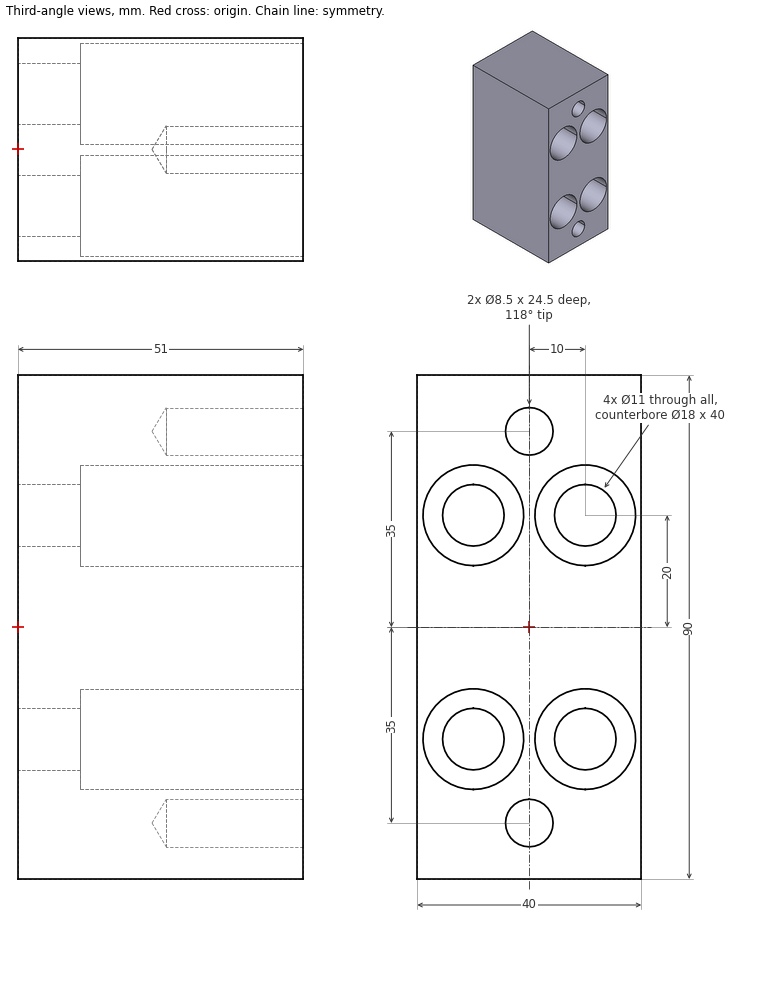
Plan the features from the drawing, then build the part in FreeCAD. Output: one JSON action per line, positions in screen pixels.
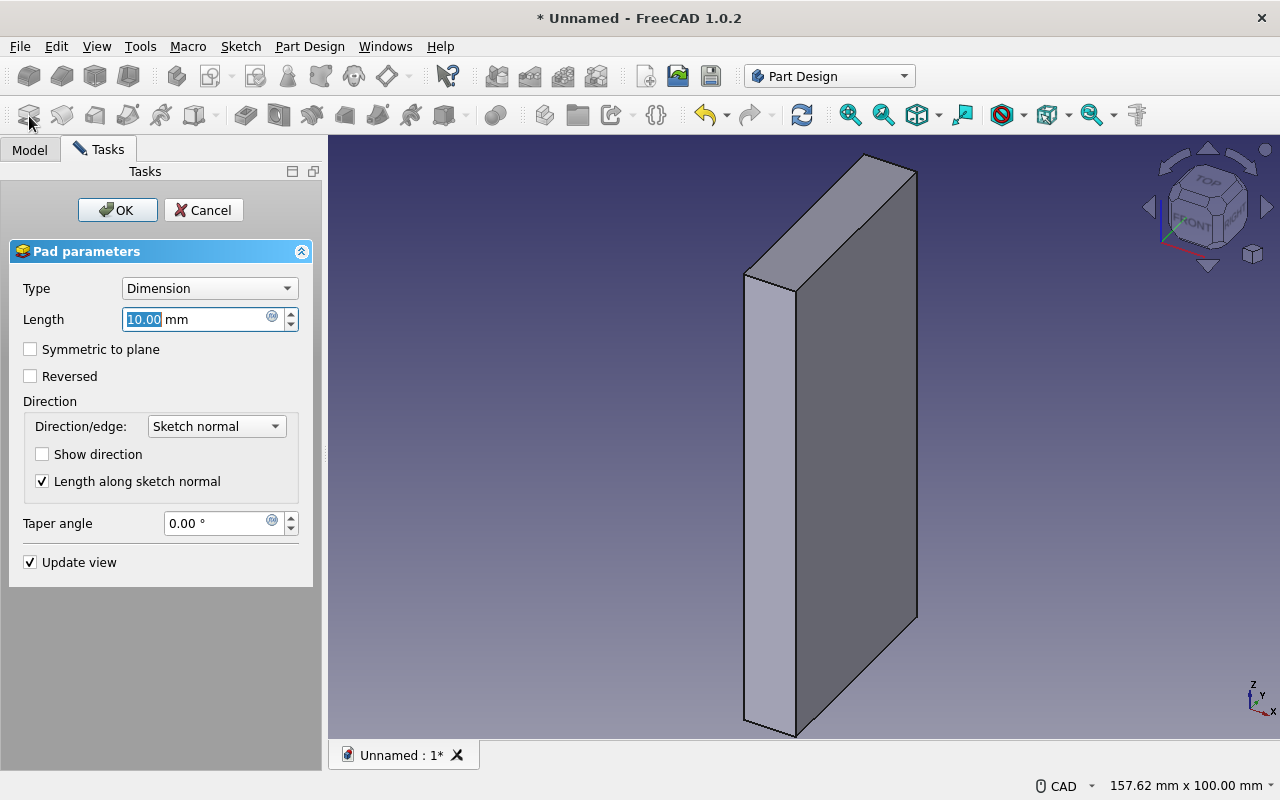
{"action": "type", "text": "51"}
{"action": "key", "text": "Tab"}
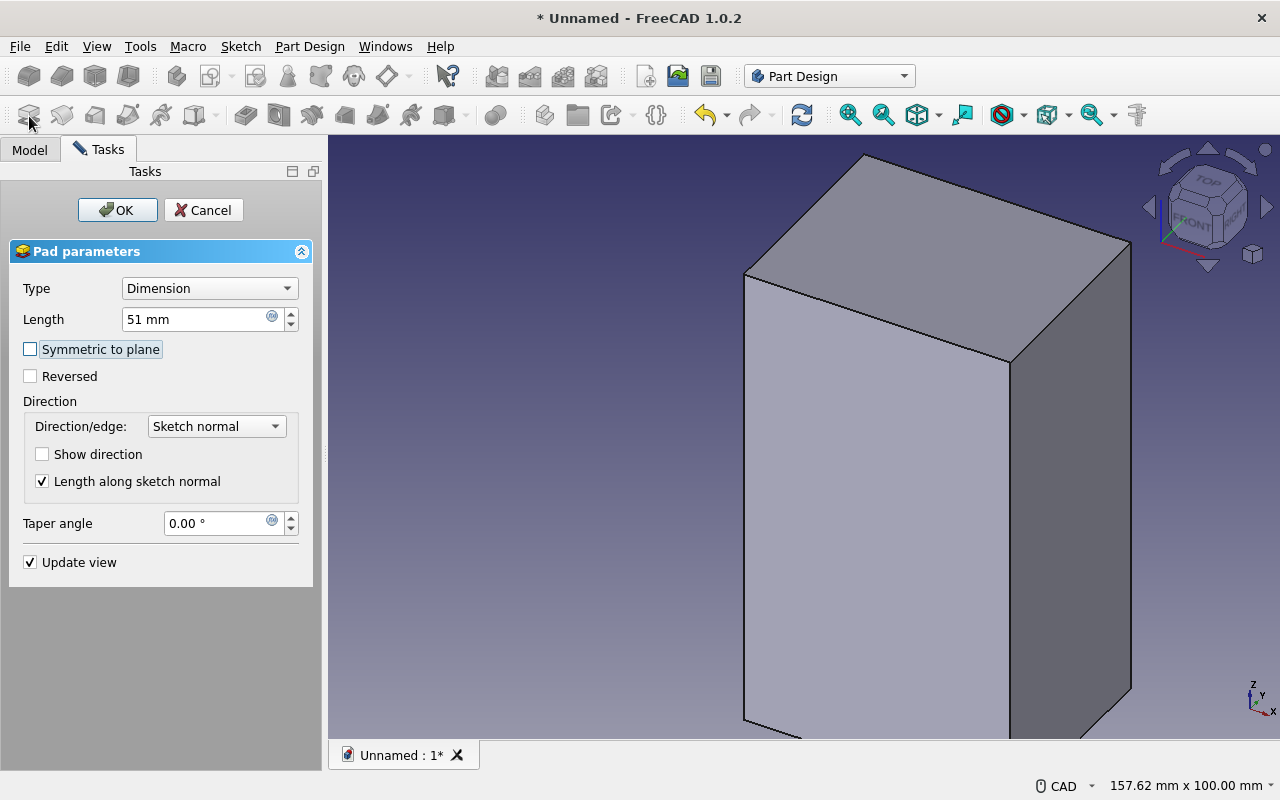
{"action": "left_click", "coordinate": [118, 210]}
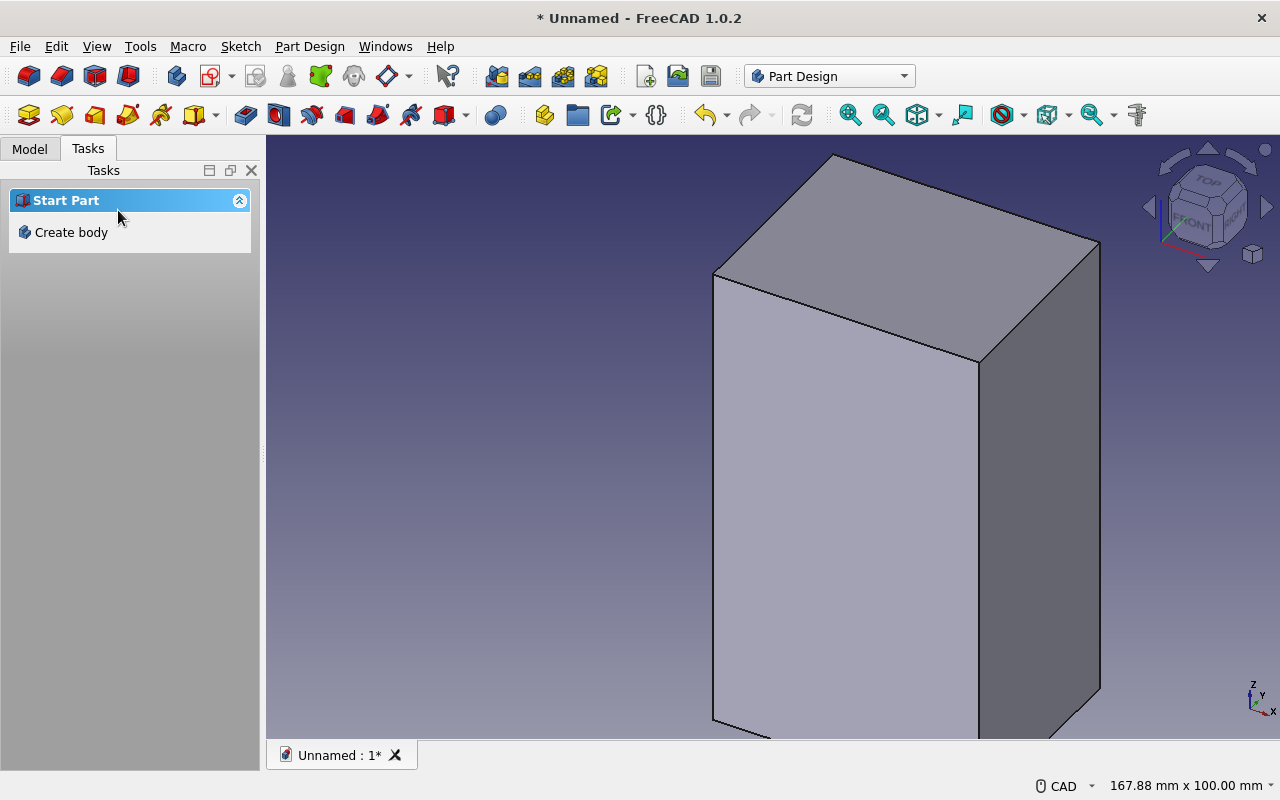
{"action": "left_click", "coordinate": [851, 116]}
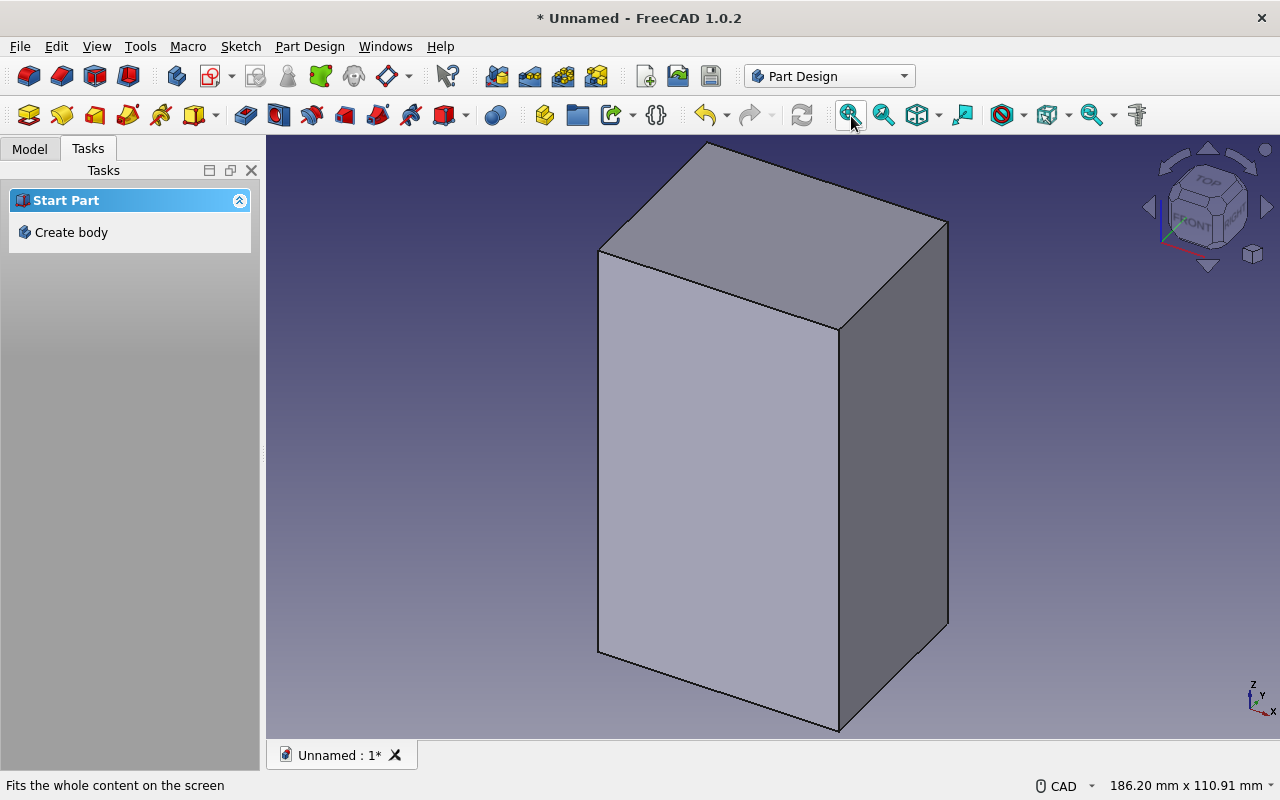
{"action": "left_click", "coordinate": [893, 533]}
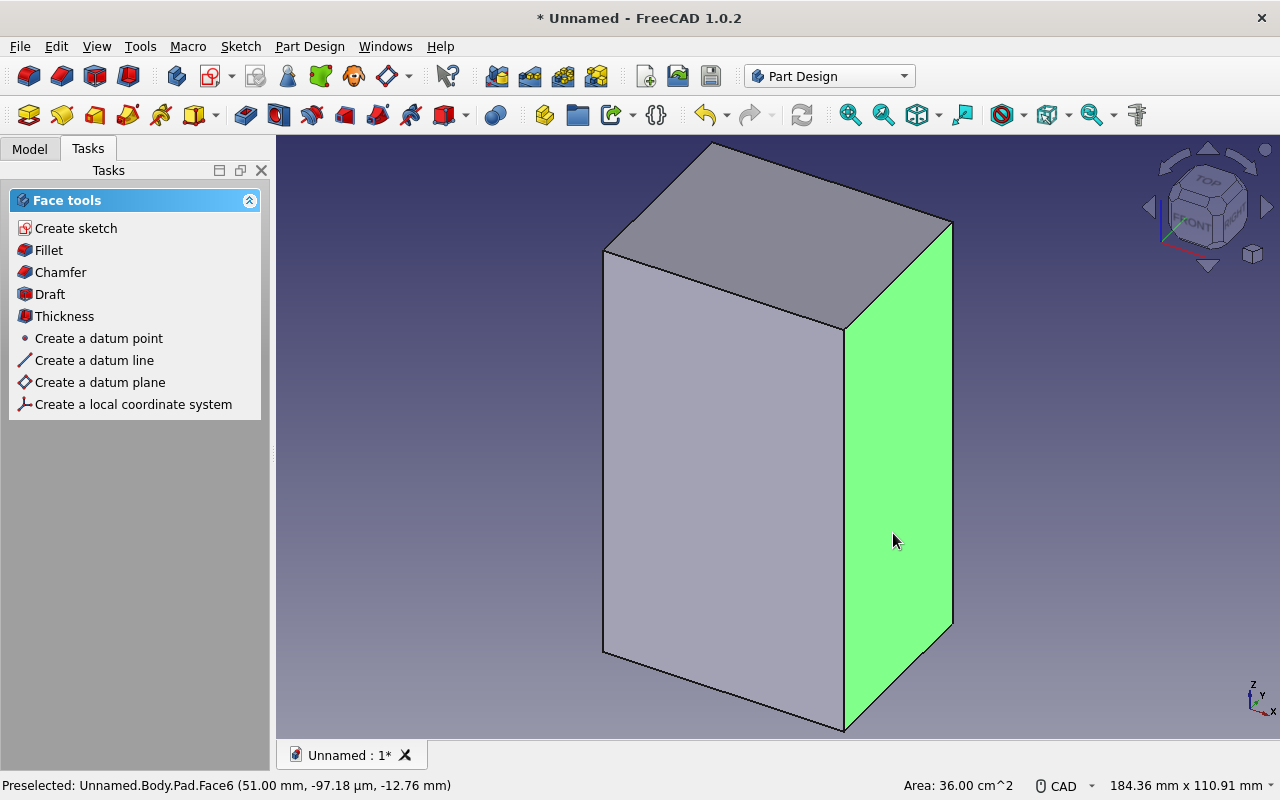
{"action": "left_click", "coordinate": [210, 76]}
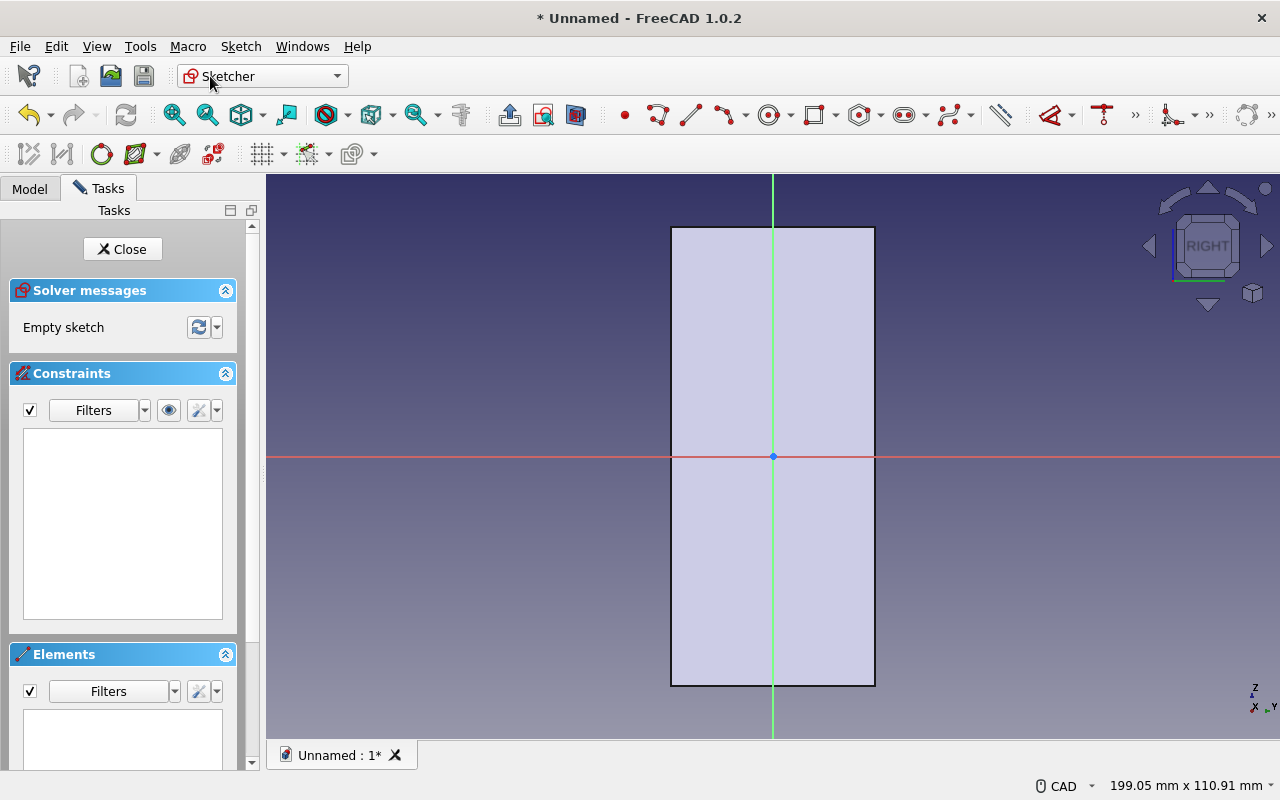
{"action": "scroll", "coordinate": [912, 456], "scroll_direction": "up", "scroll_amount": 2}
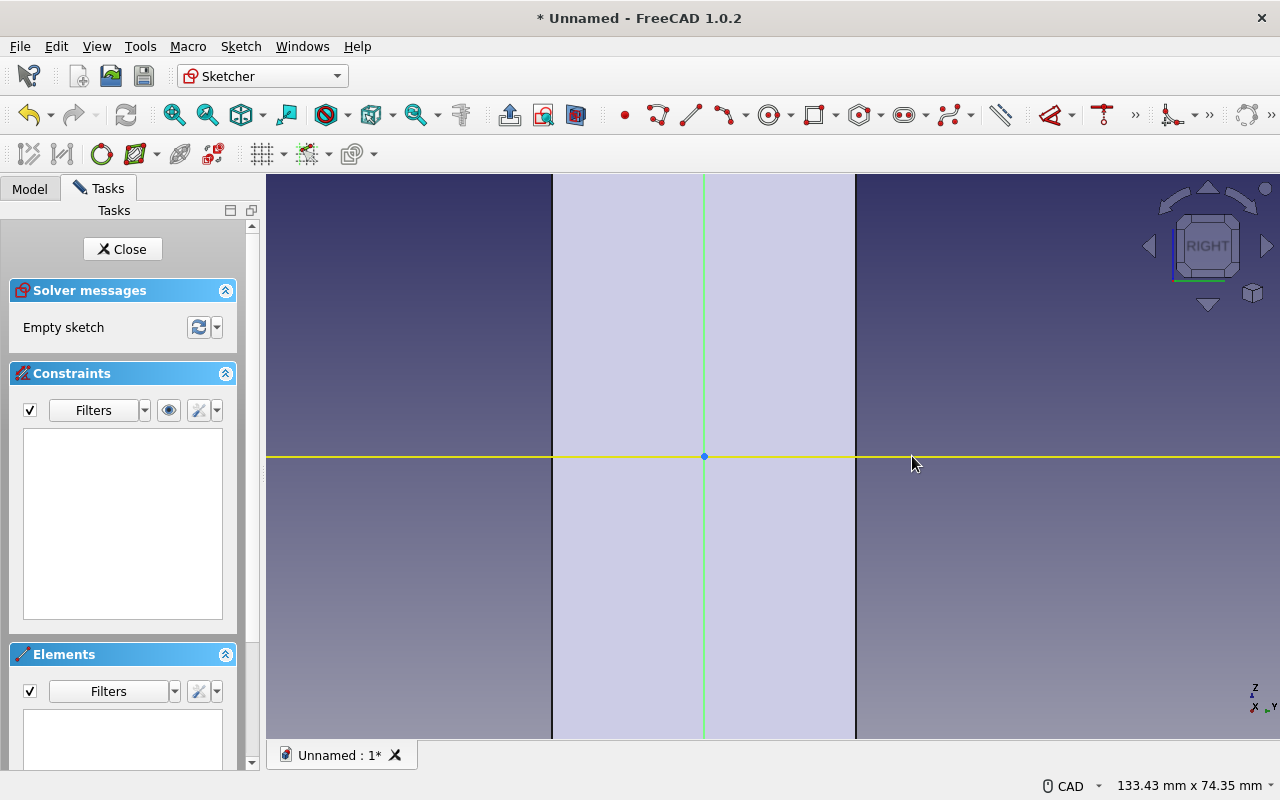
{"action": "left_click", "coordinate": [768, 116]}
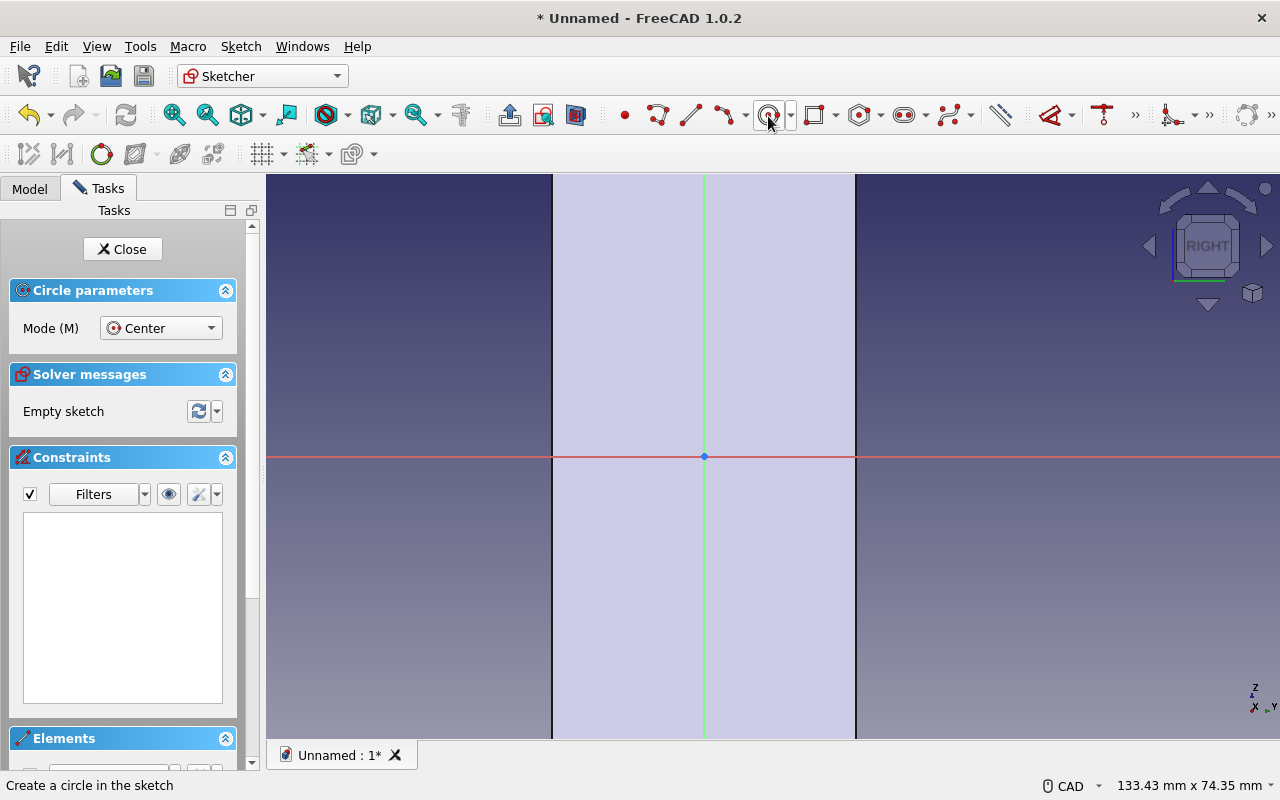
{"action": "left_click", "coordinate": [780, 305]}
{"action": "mouse_move", "coordinate": [810, 275]}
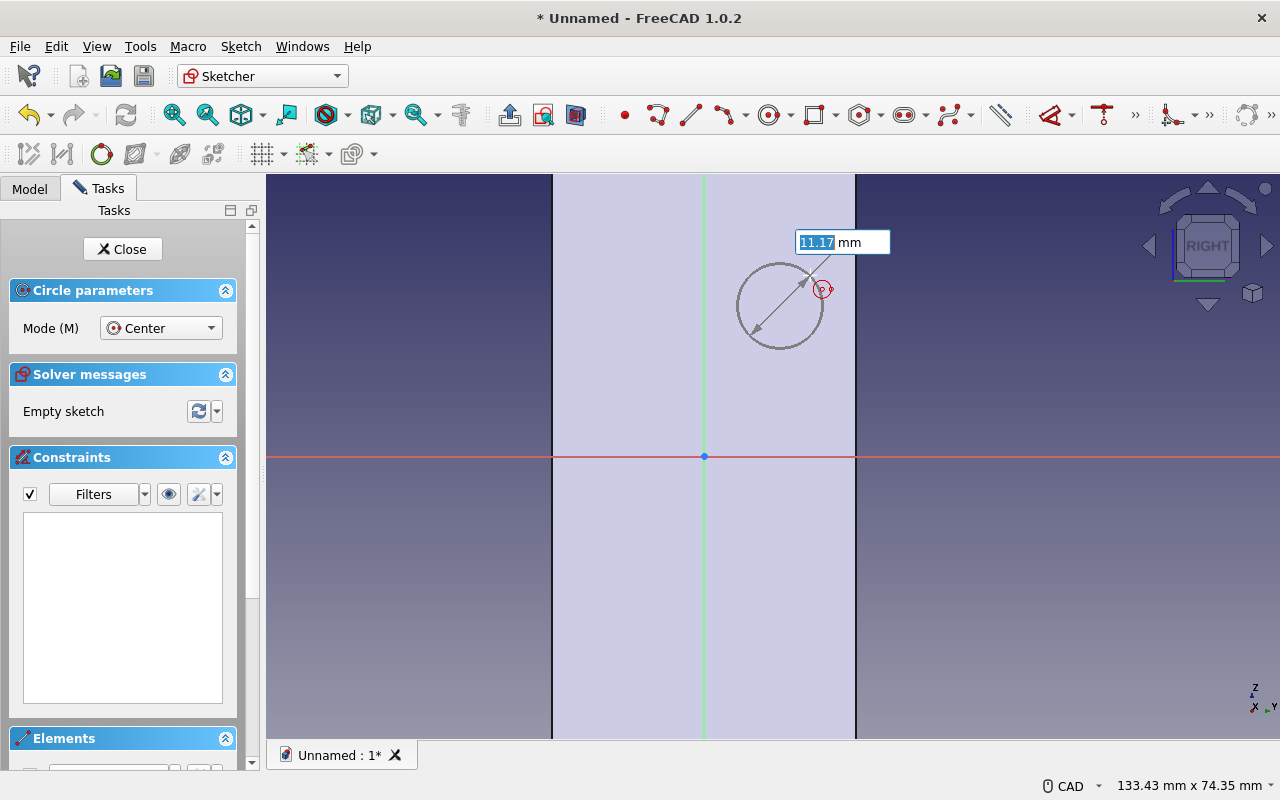
{"action": "type", "text": "11"}
{"action": "key", "text": "Return"}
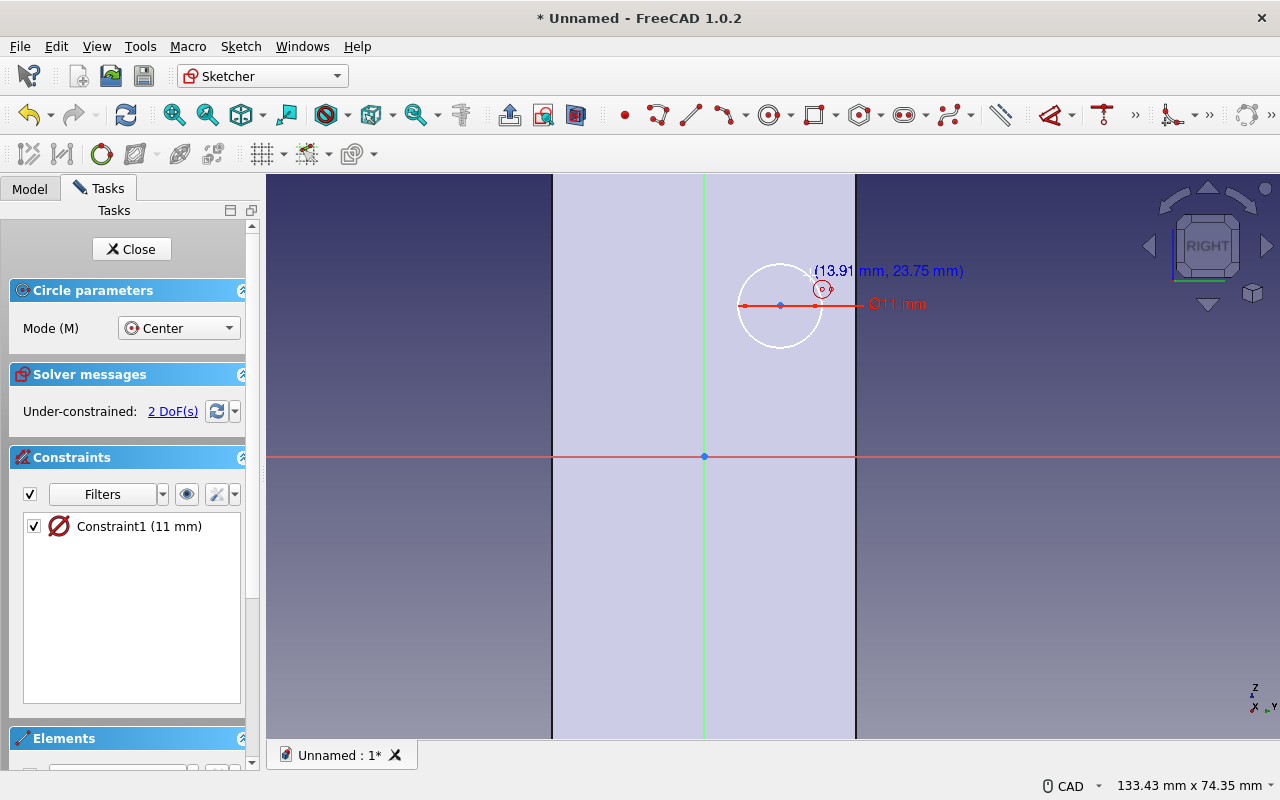
{"action": "left_click", "coordinate": [780, 608]}
{"action": "mouse_move", "coordinate": [810, 579]}